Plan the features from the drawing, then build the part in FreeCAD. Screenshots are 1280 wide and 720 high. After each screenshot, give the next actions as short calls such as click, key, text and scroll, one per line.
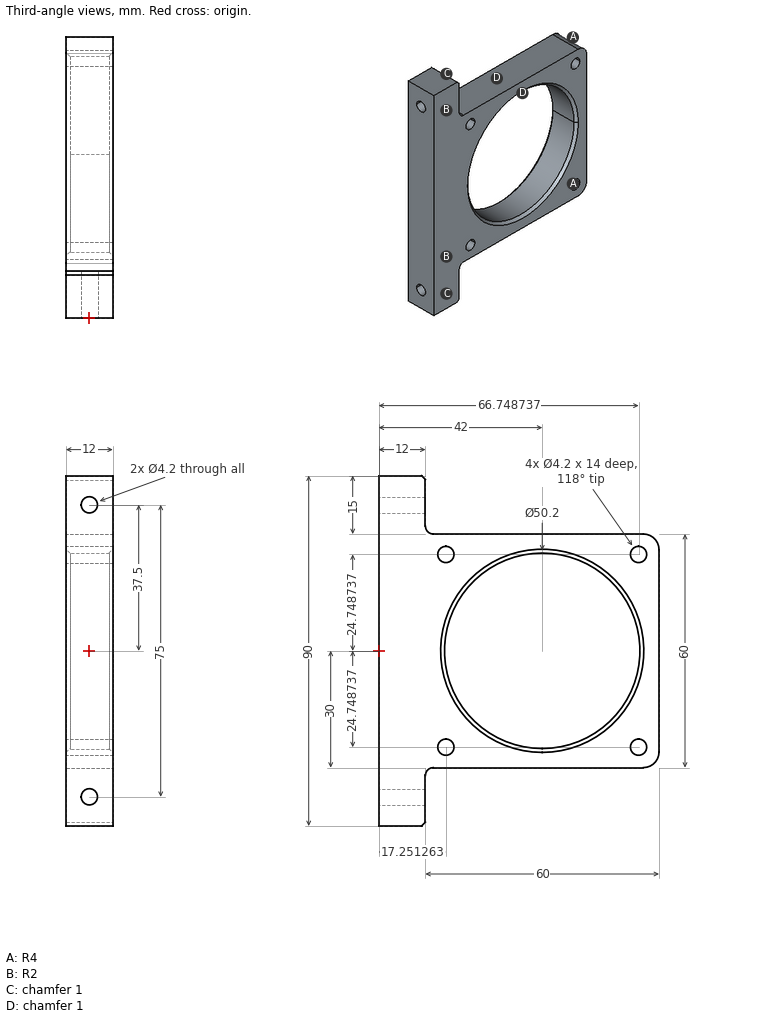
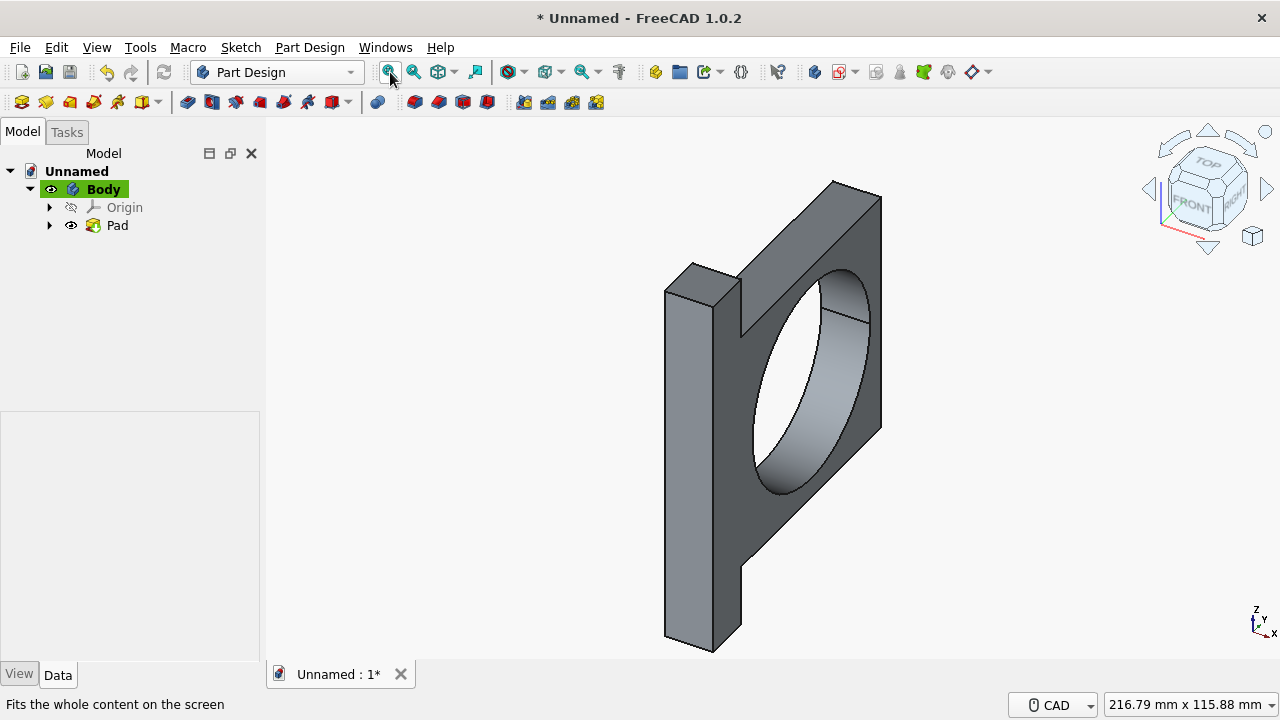
key(0)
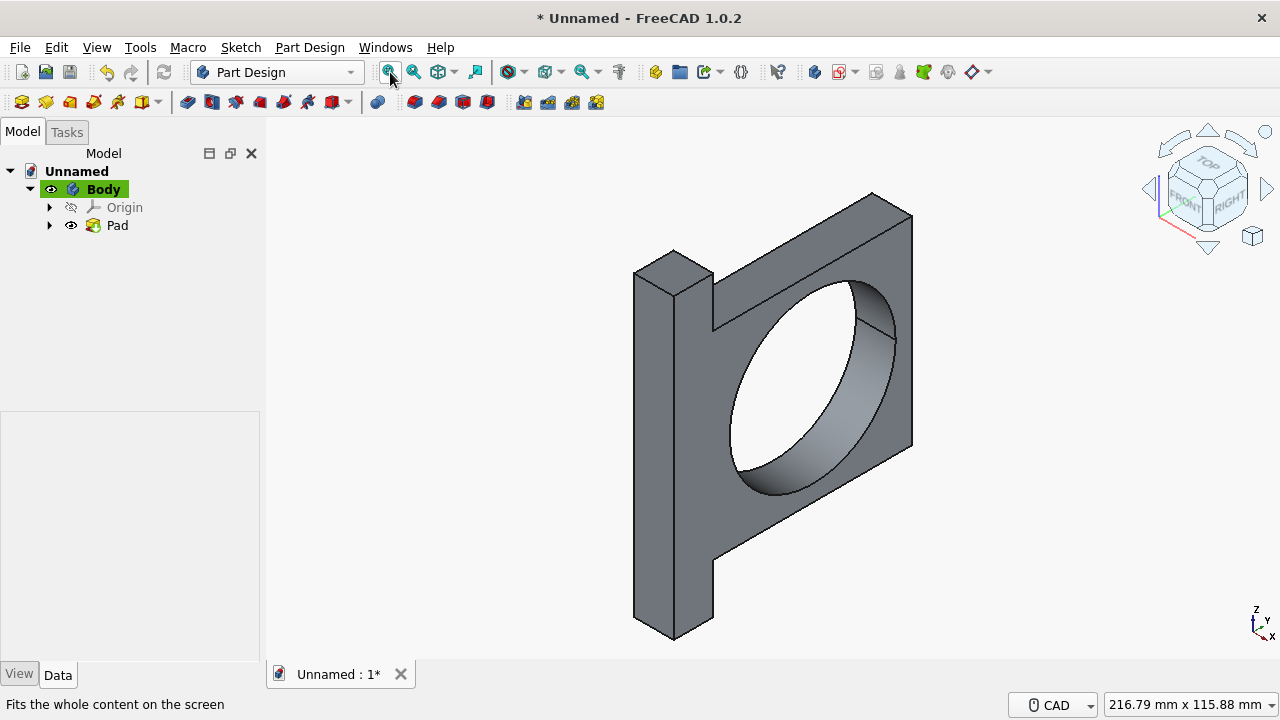
key(2)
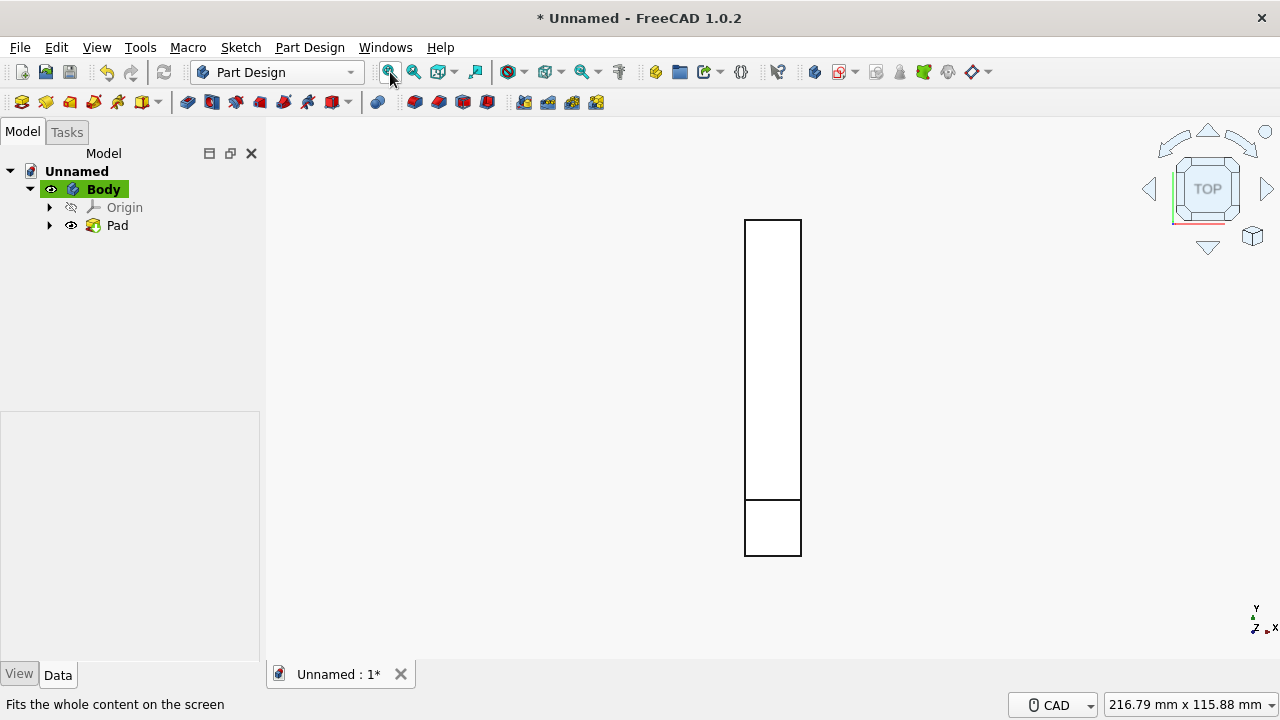
click(773, 219)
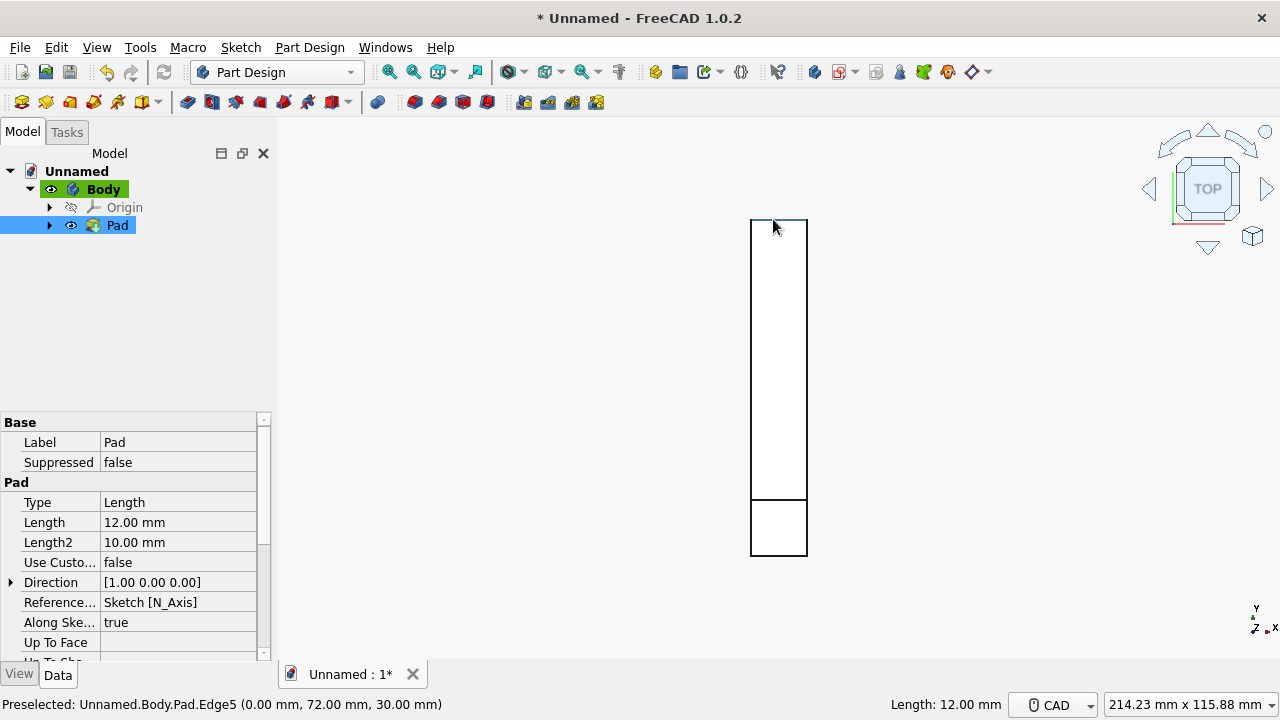
key(1)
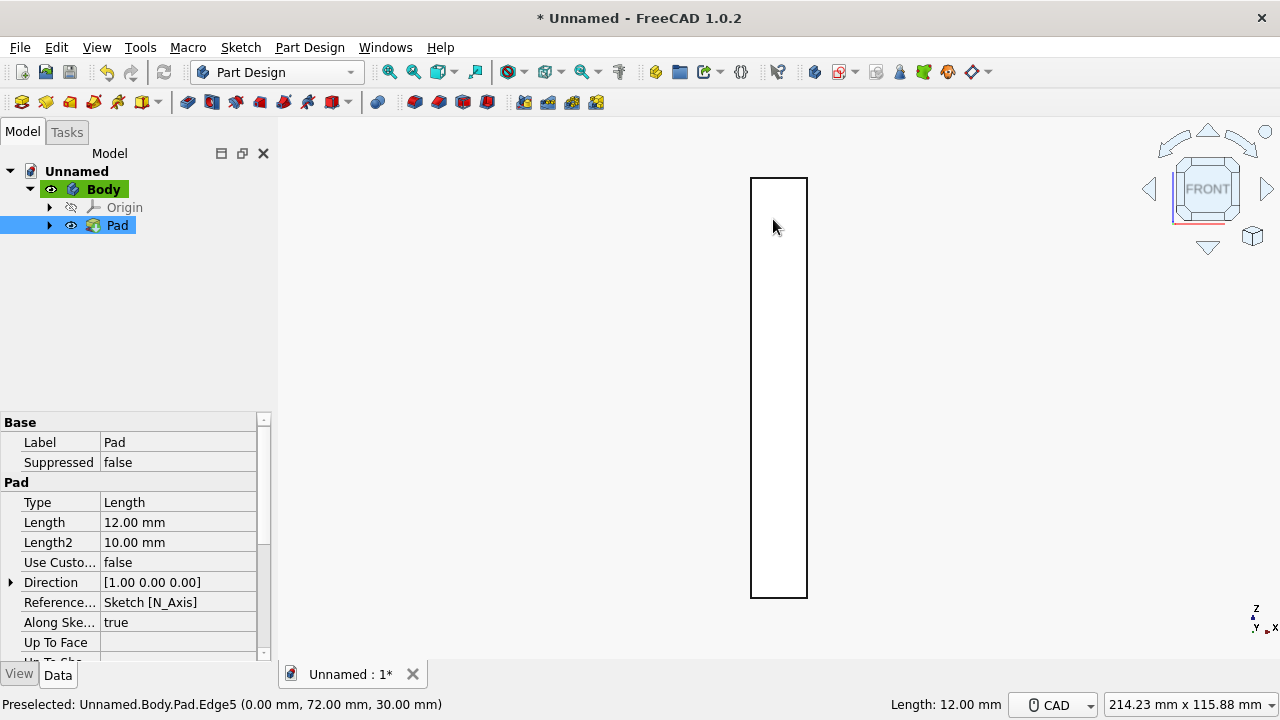
key(3)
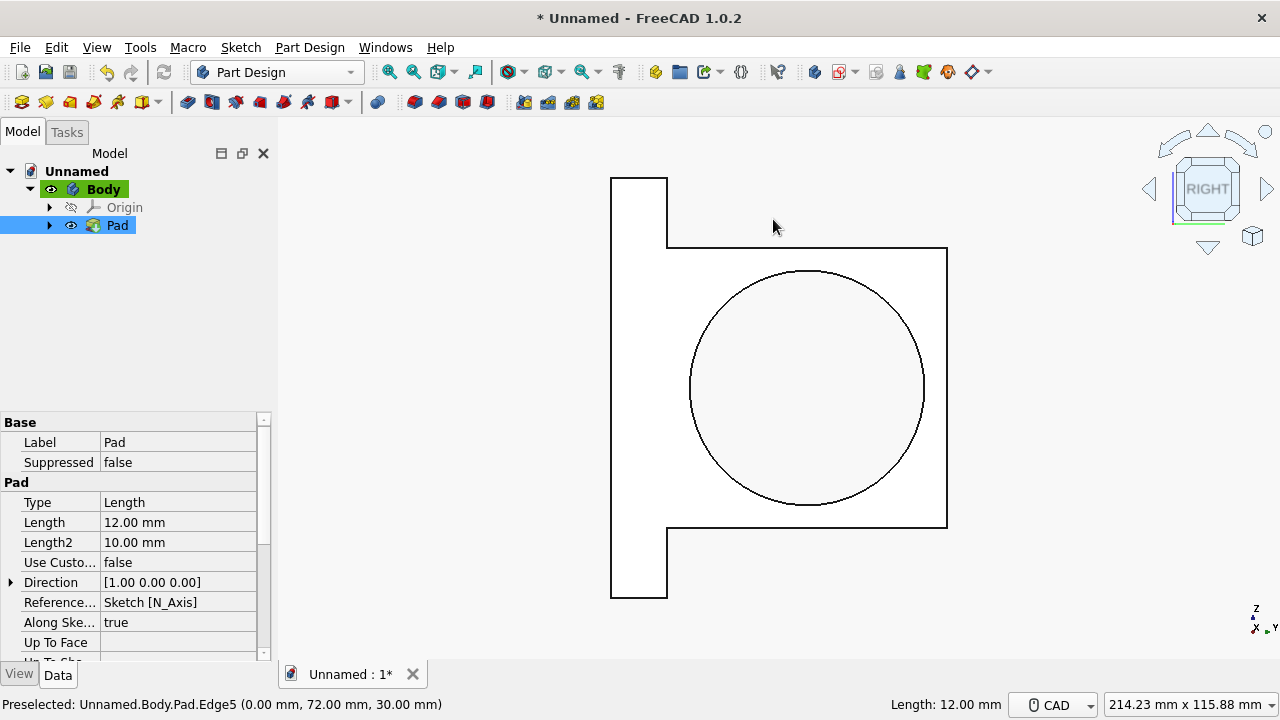
key(5)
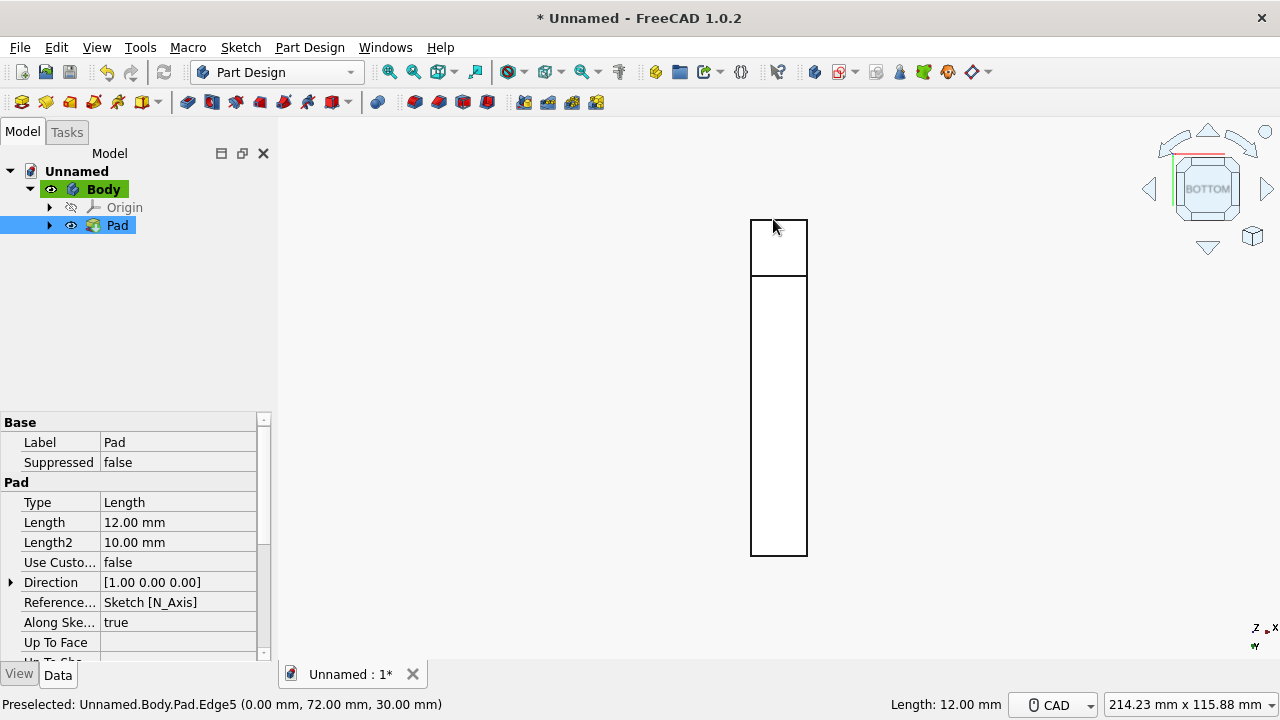
click(779, 555, ctrl)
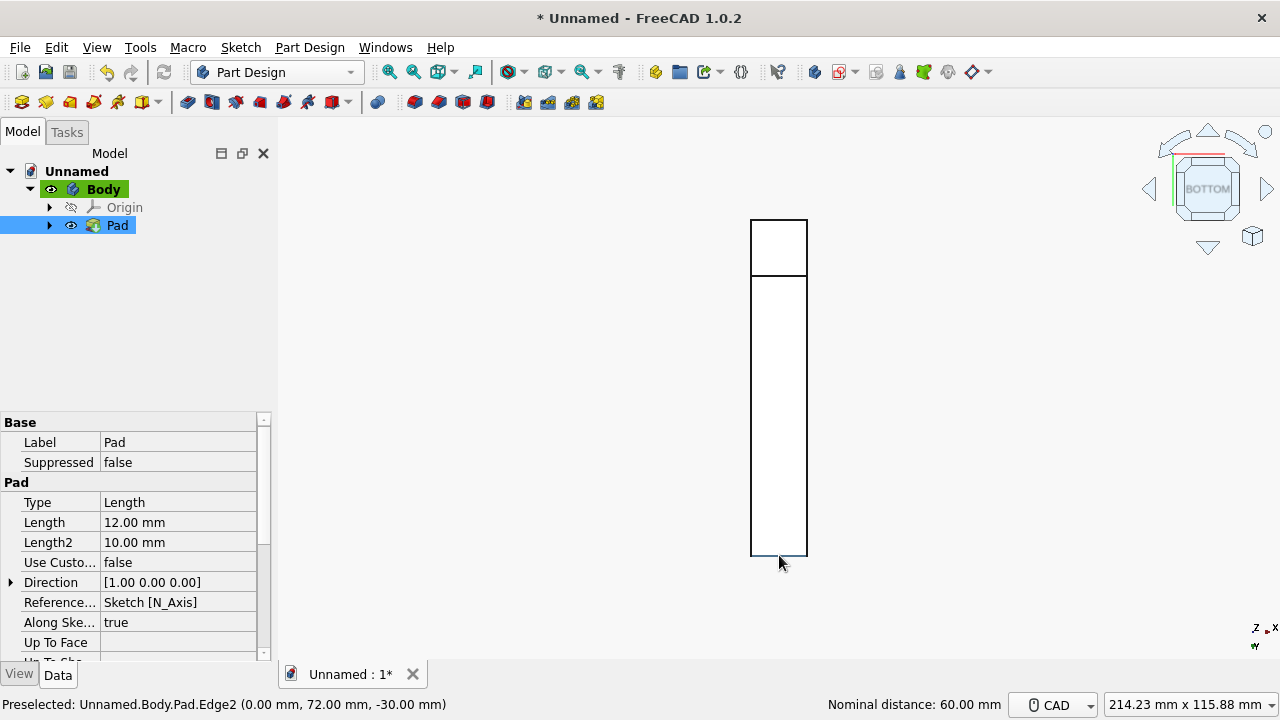
click(416, 102)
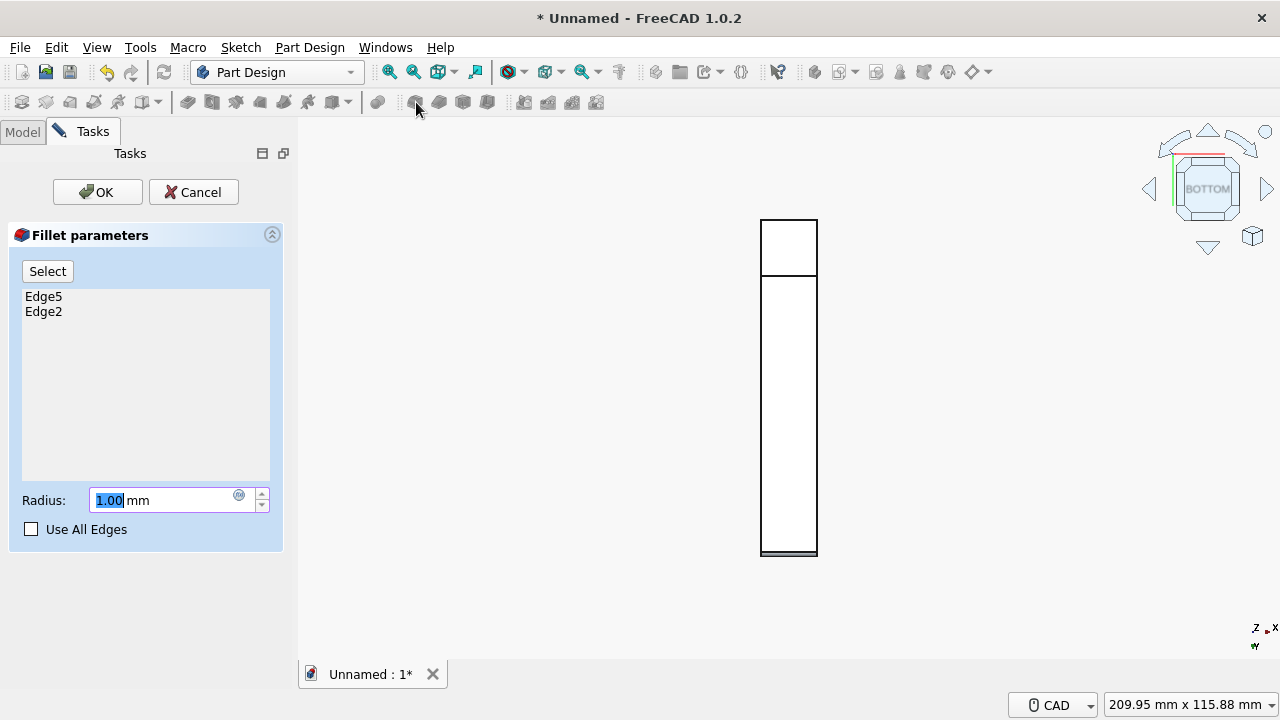
text(4)
key(Tab)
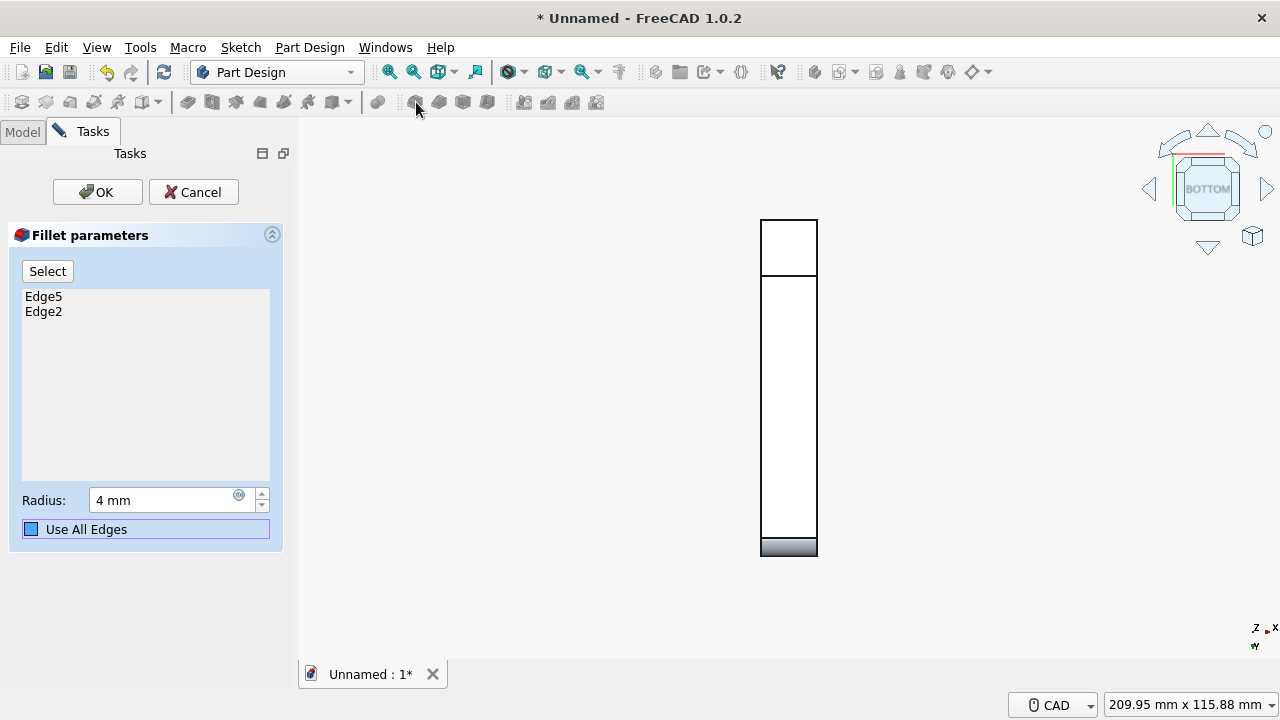
click(98, 192)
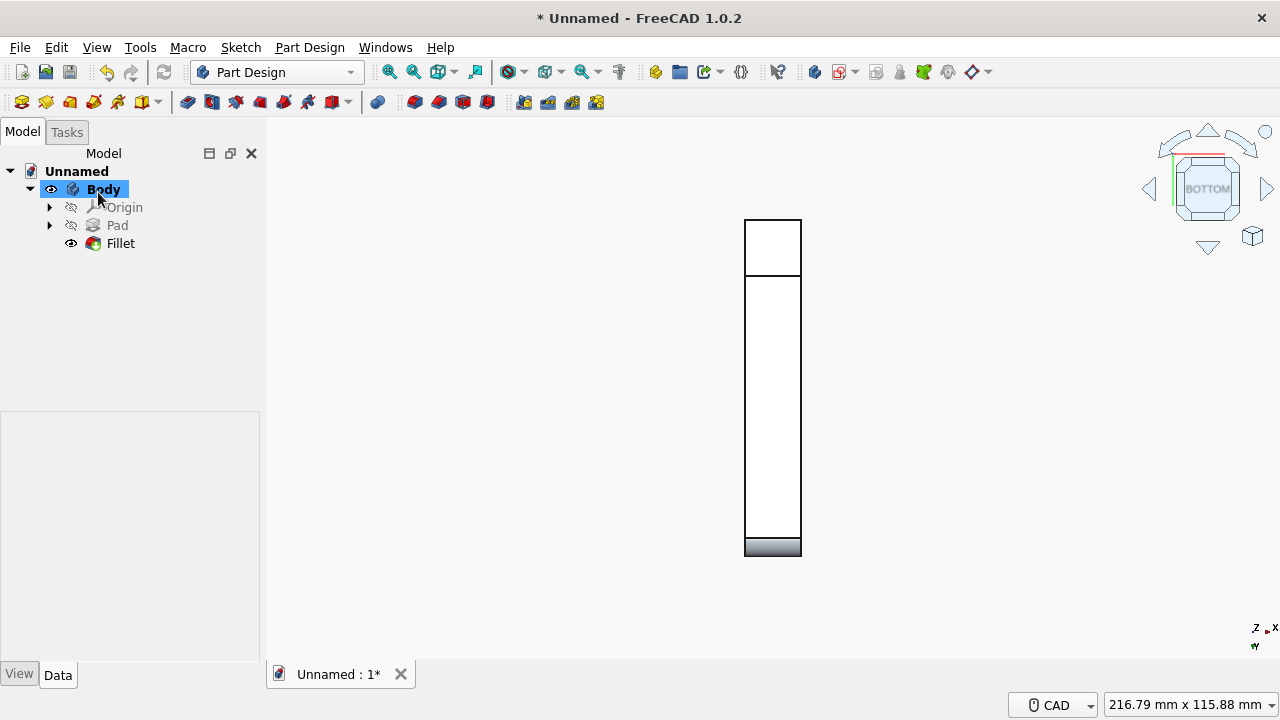
key(0)